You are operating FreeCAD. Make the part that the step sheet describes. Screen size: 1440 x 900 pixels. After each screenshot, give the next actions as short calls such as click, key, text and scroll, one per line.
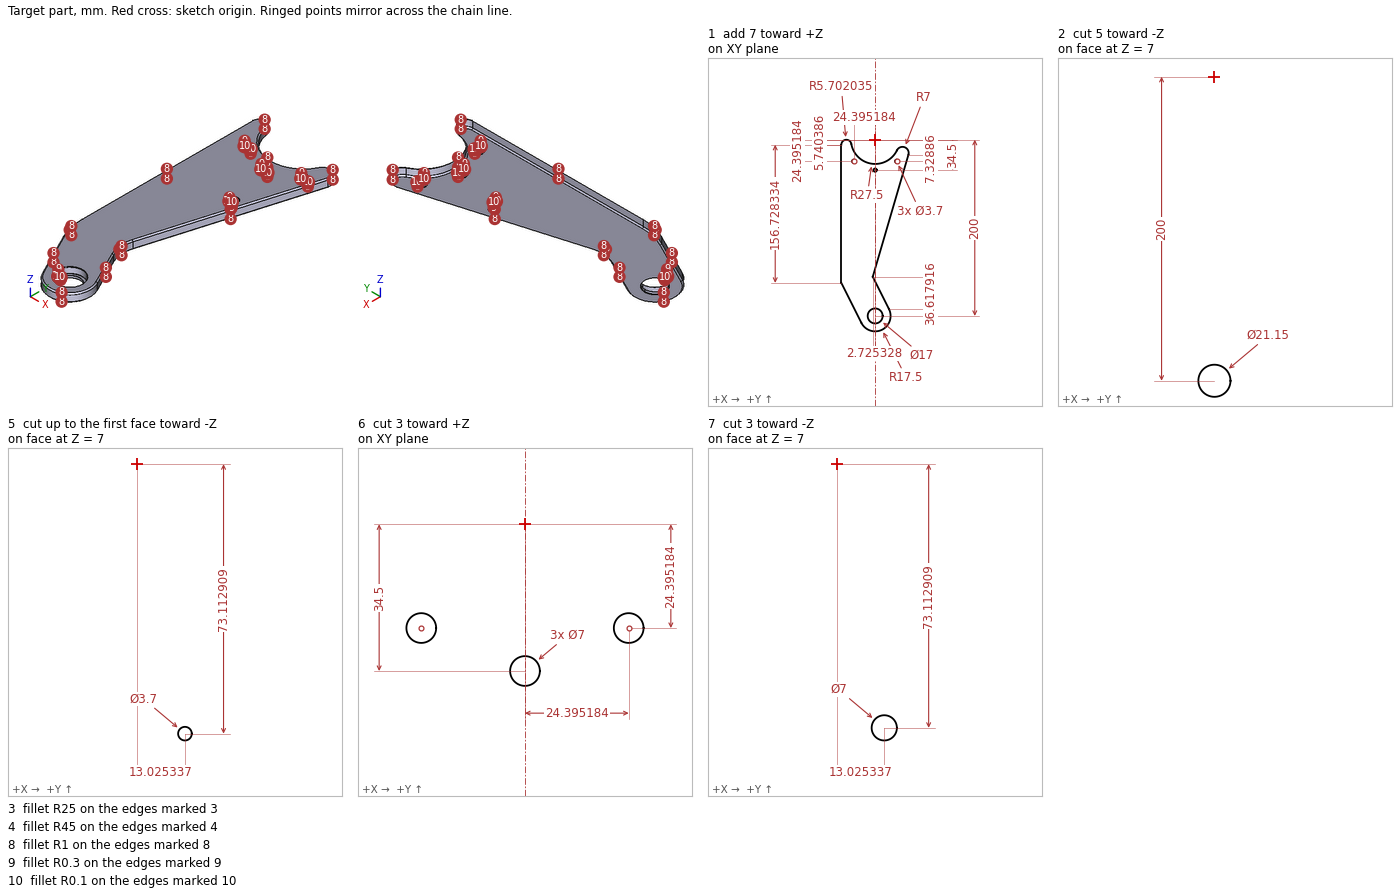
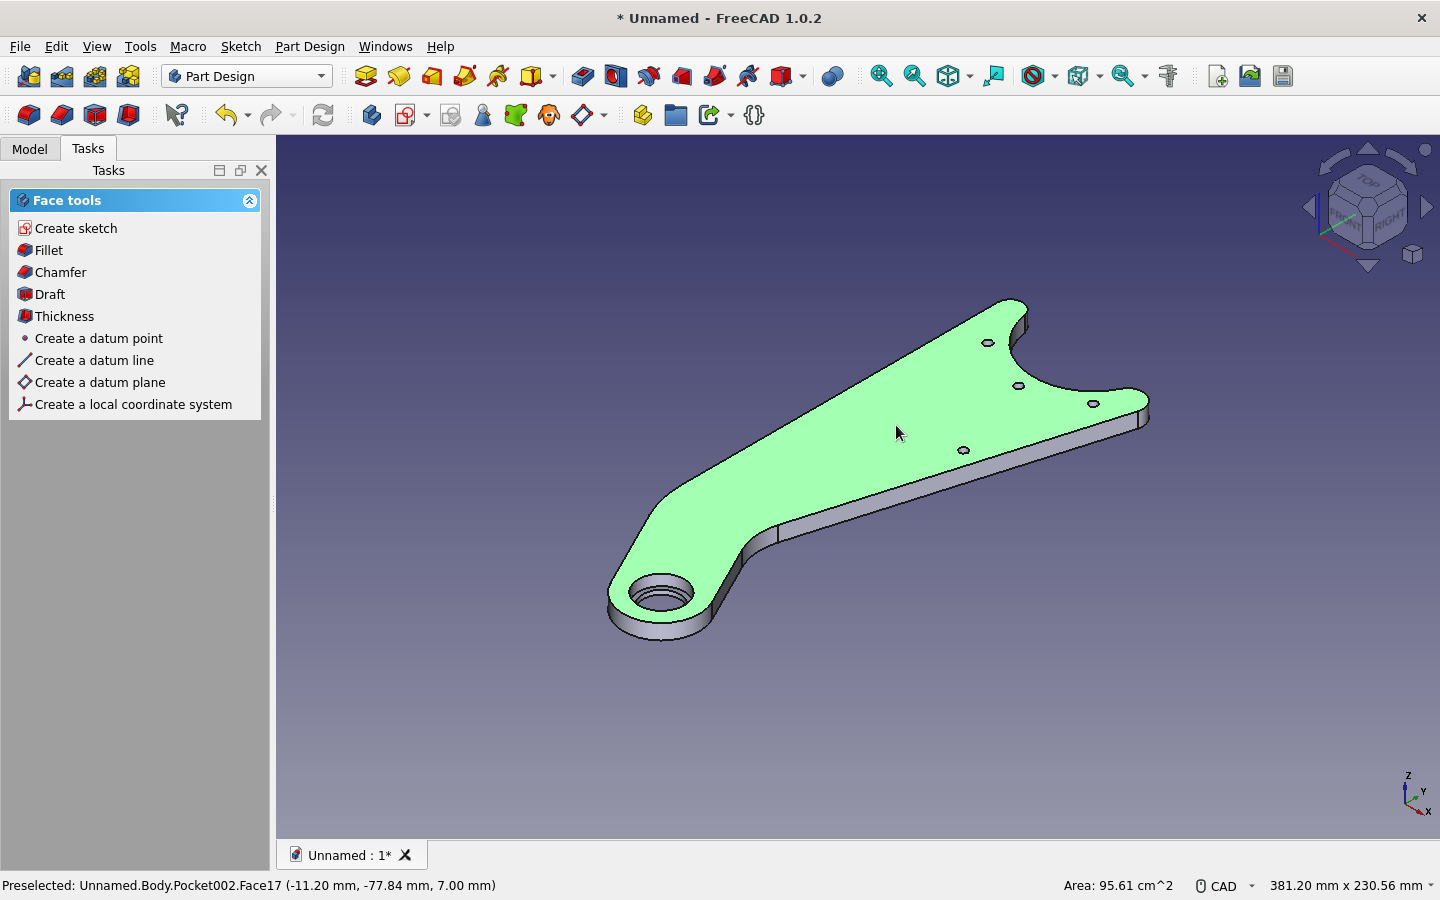
click(404, 116)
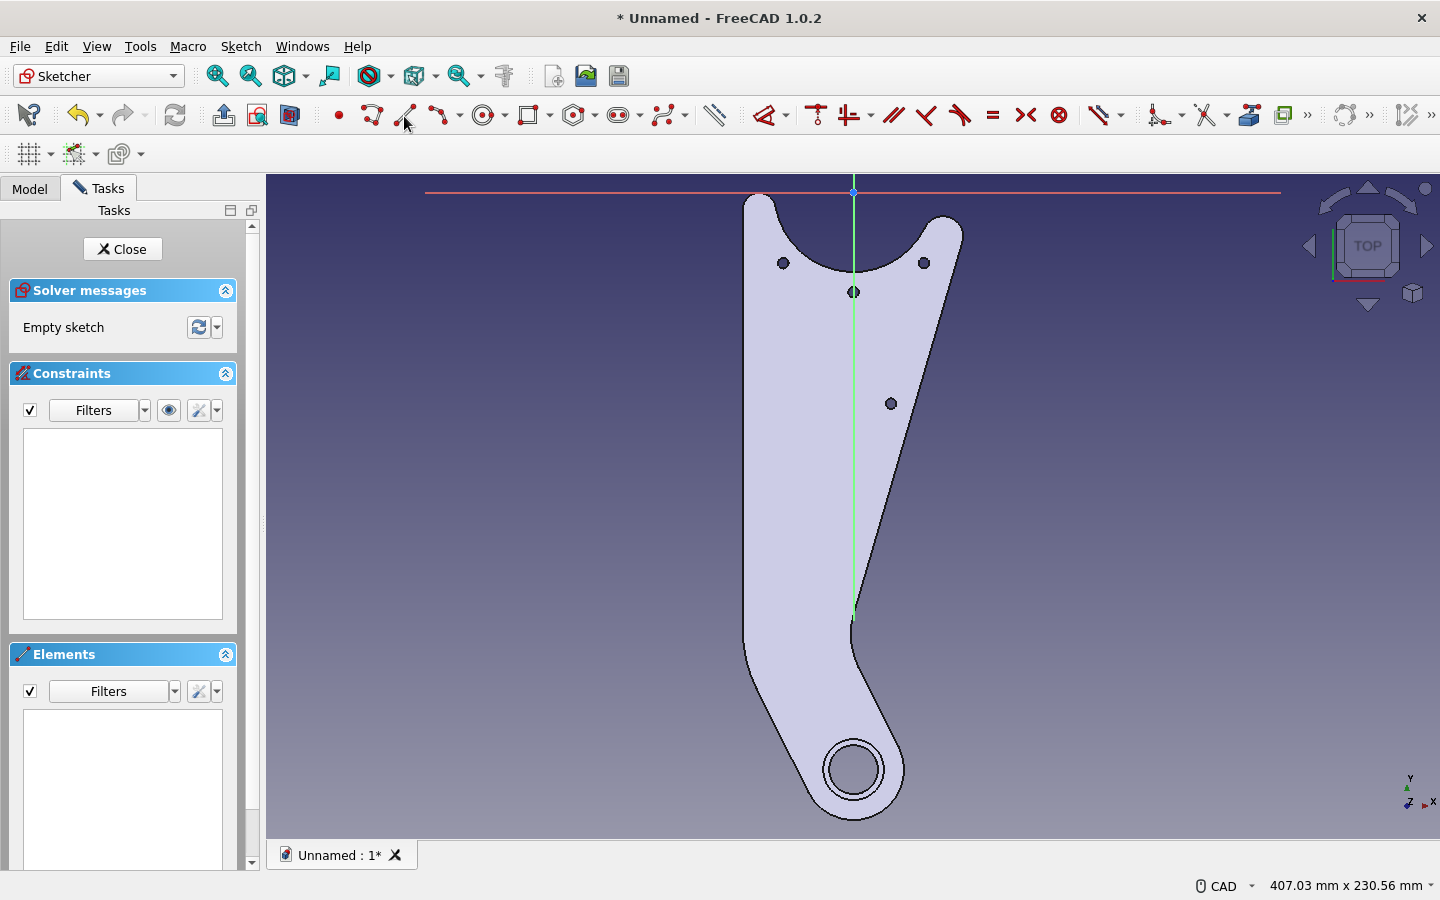
scroll(897, 398, up, 15)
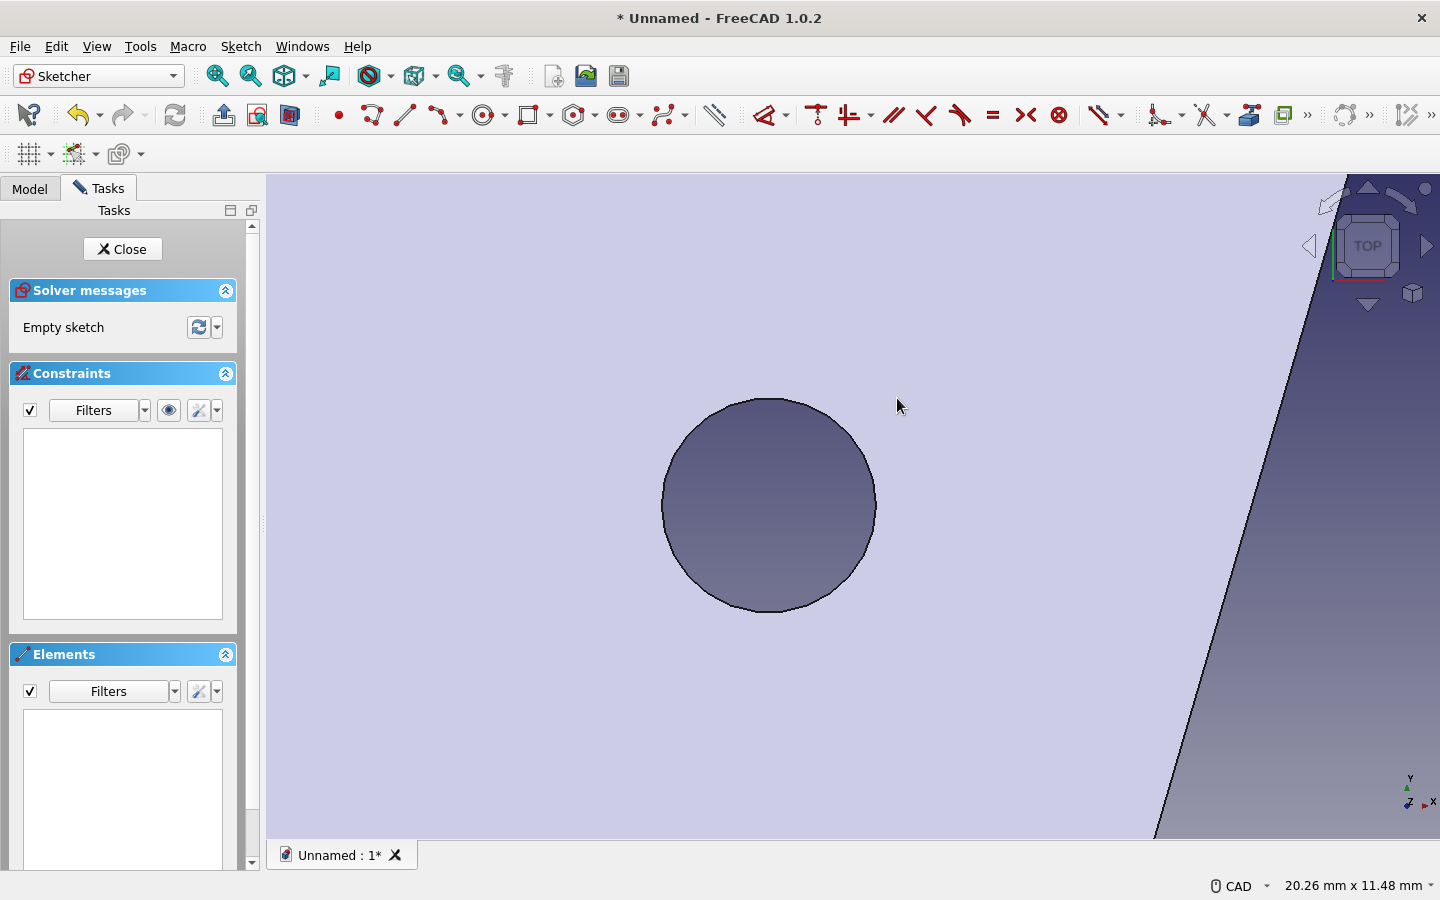
click(482, 116)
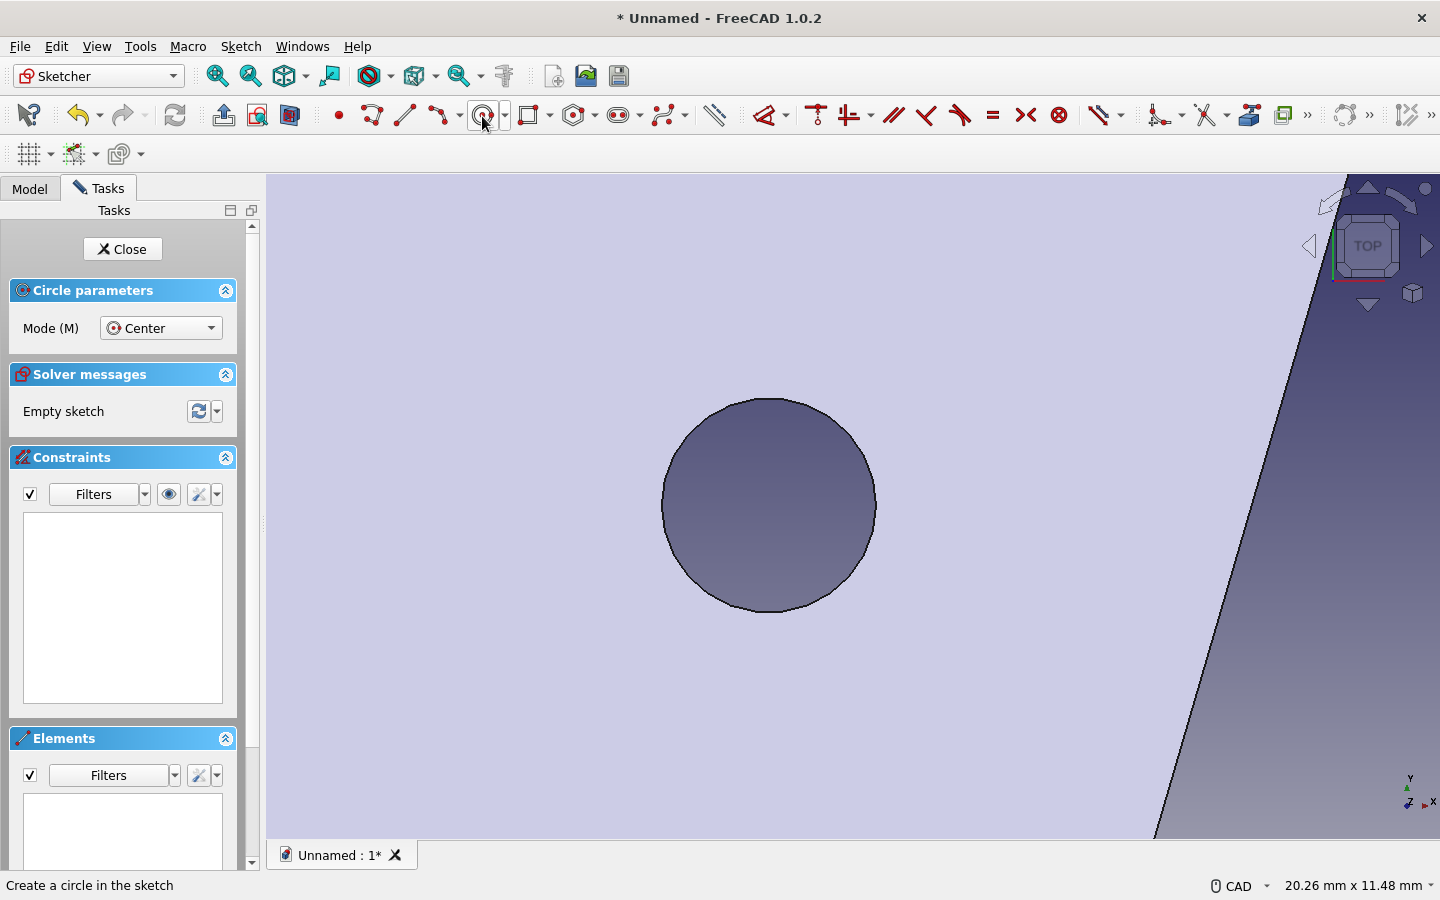
click(769, 505)
click(912, 362)
key(Escape)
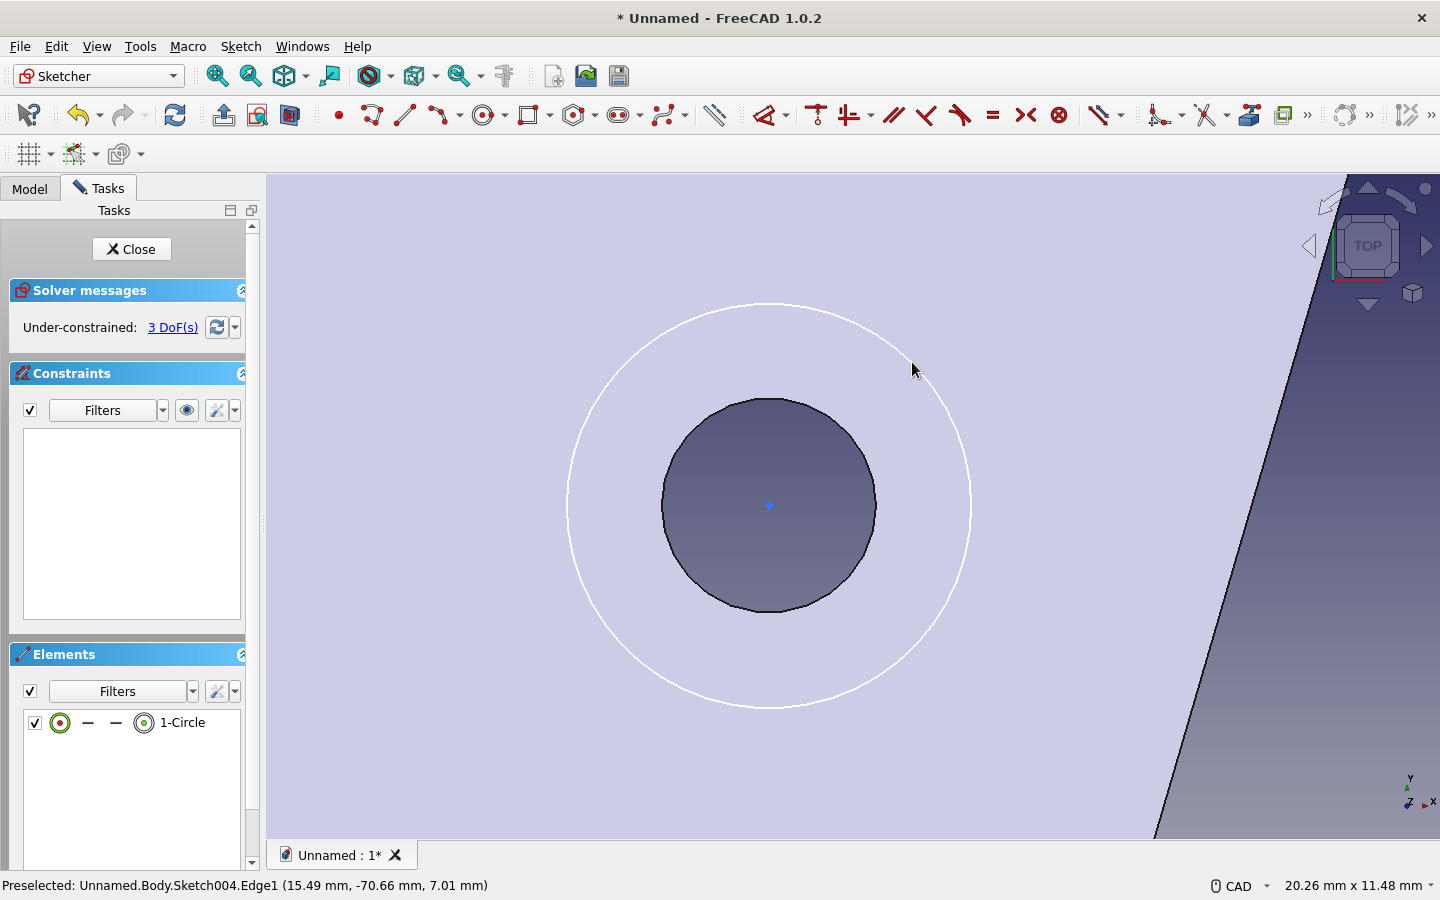
click(764, 116)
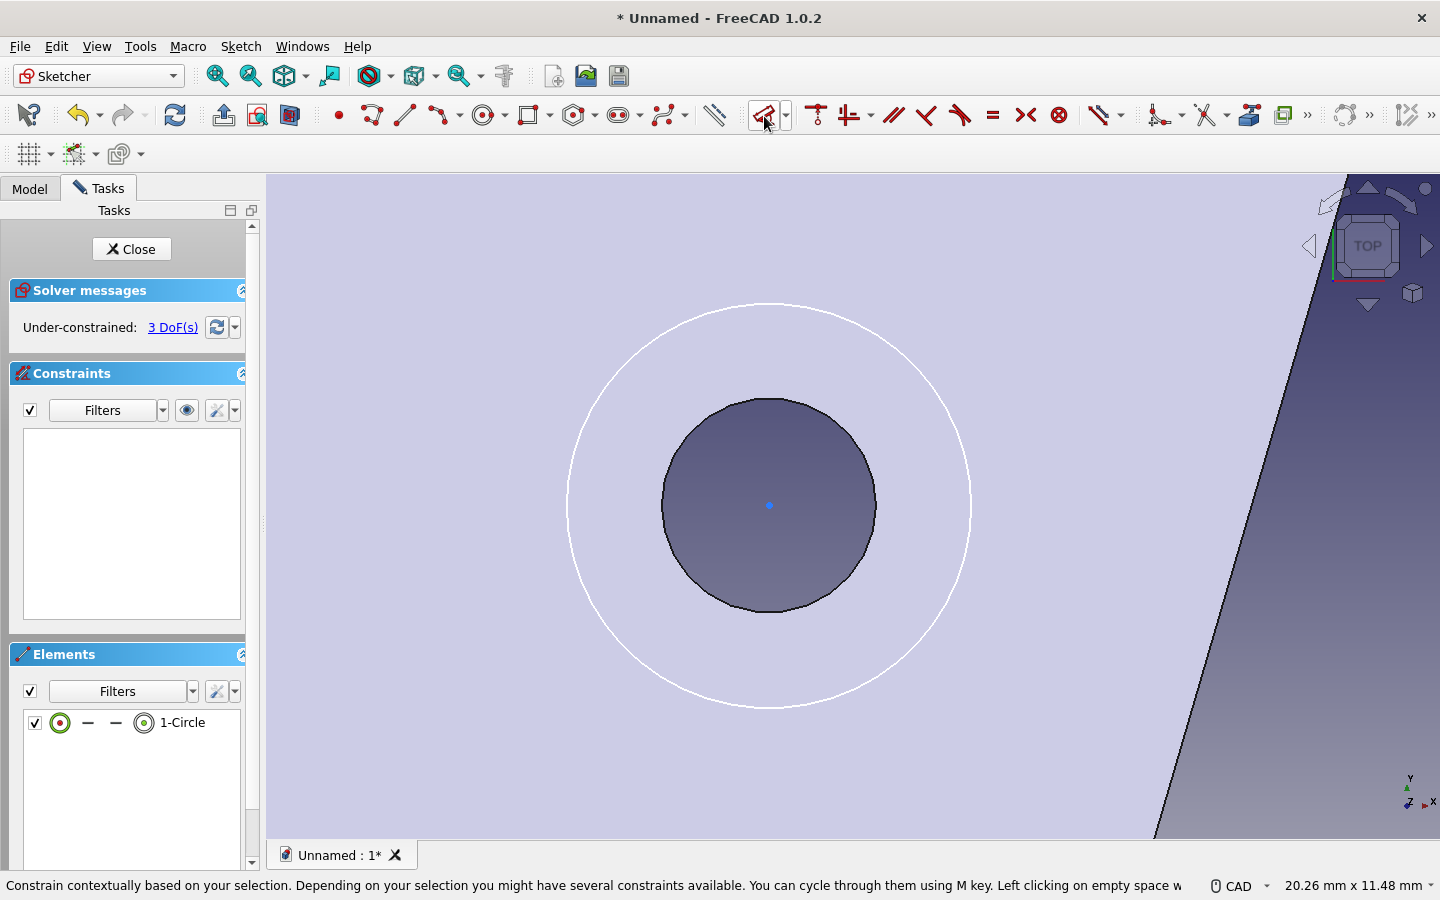
click(912, 363)
click(935, 340)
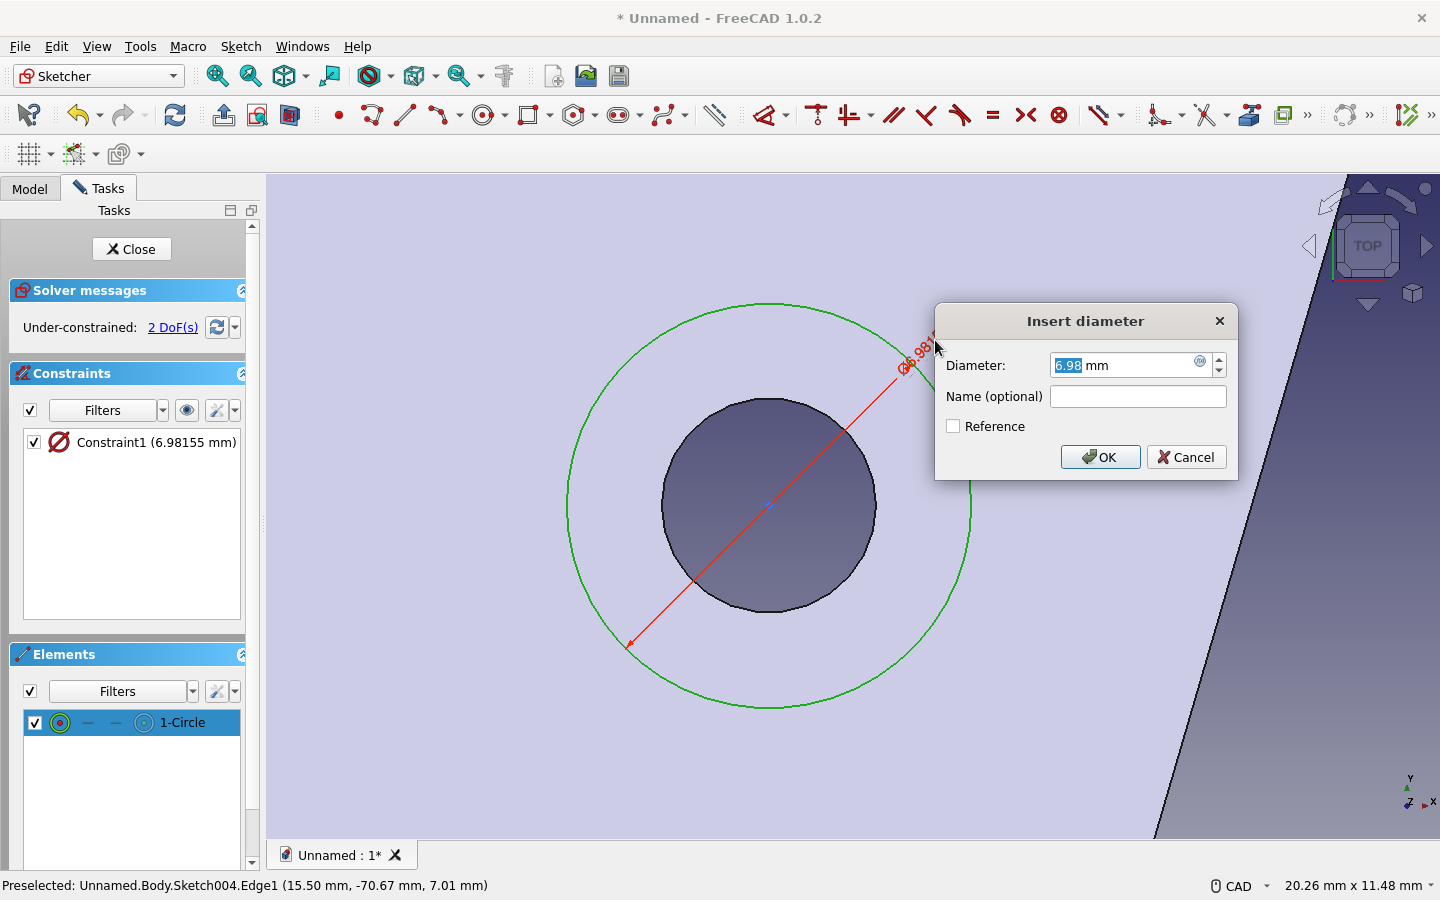
text(7)
key(Return)